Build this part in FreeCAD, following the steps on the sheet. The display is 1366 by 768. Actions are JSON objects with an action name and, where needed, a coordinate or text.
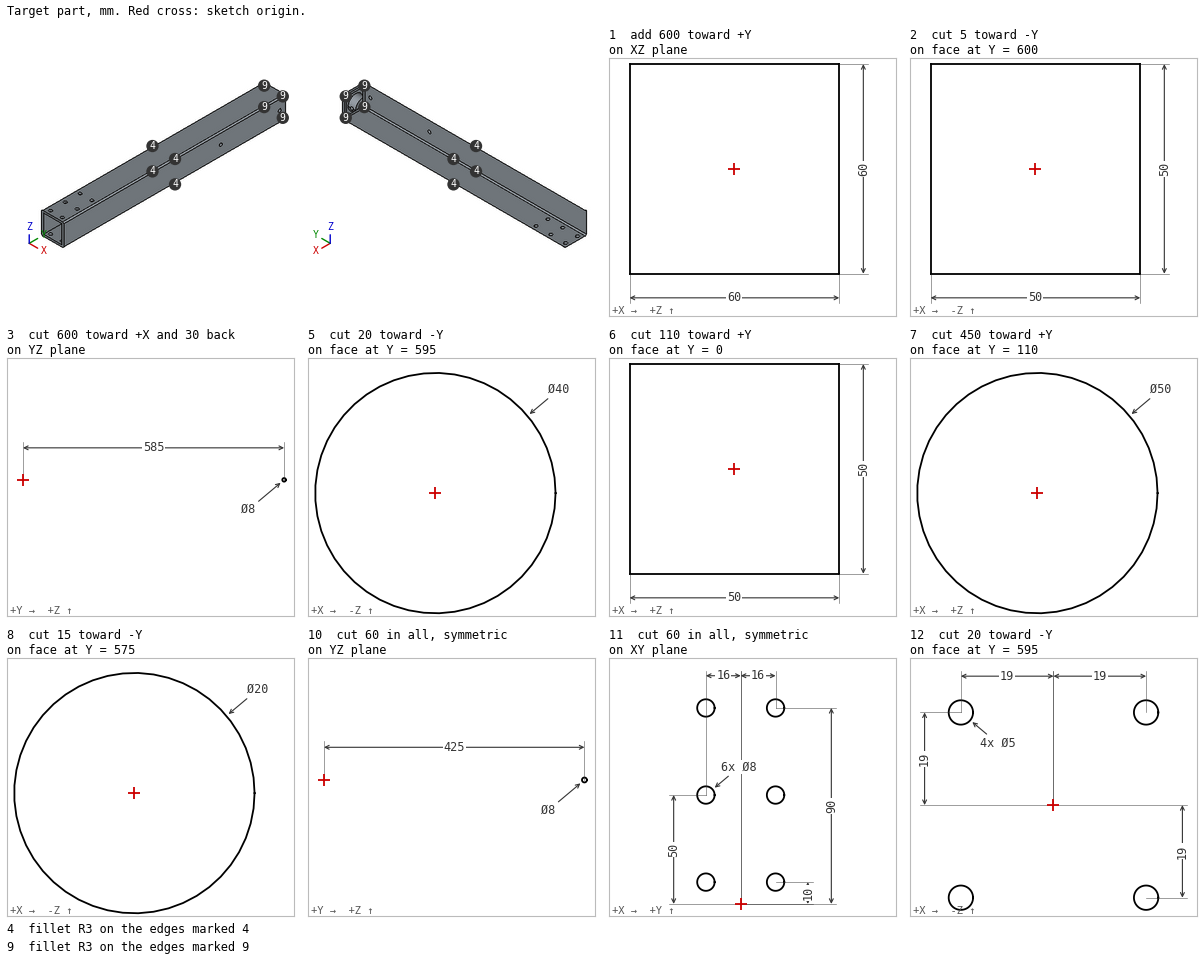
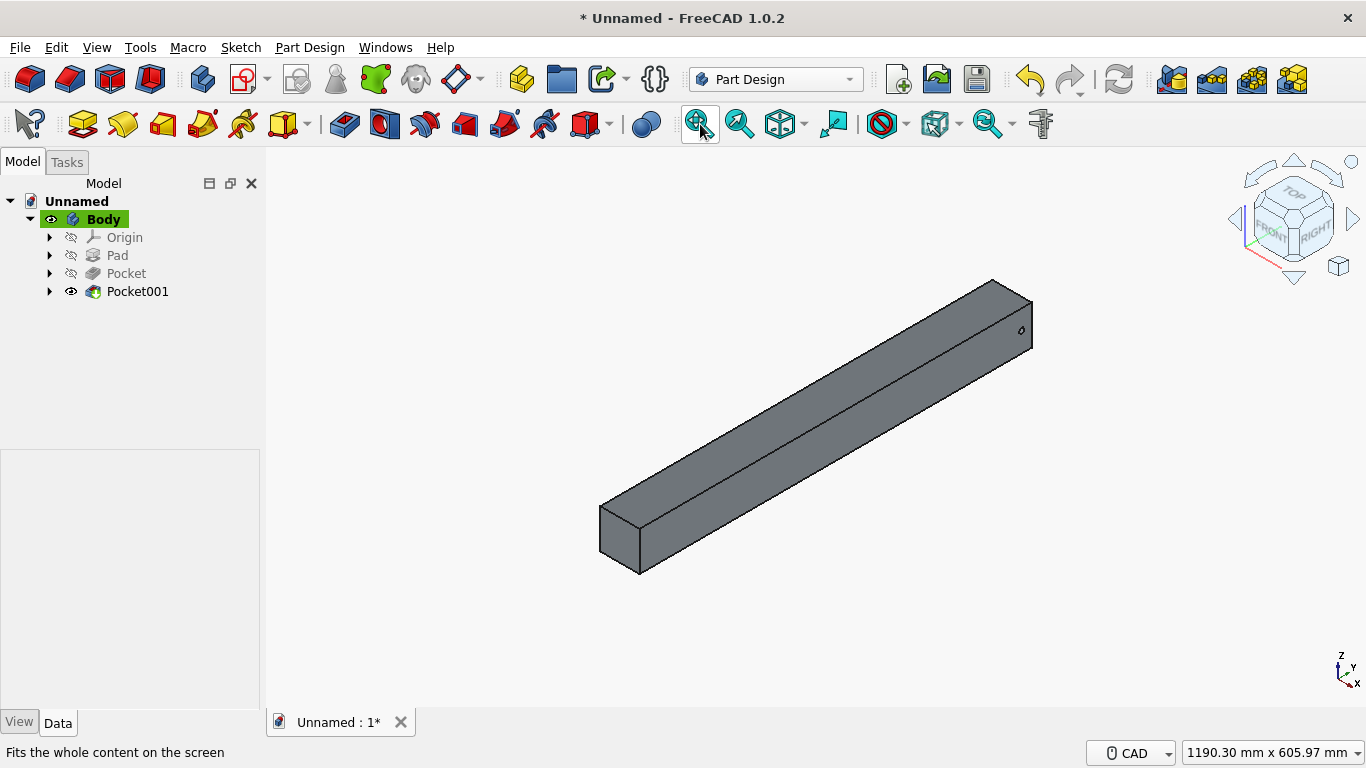
{"action": "left_click", "coordinate": [836, 415]}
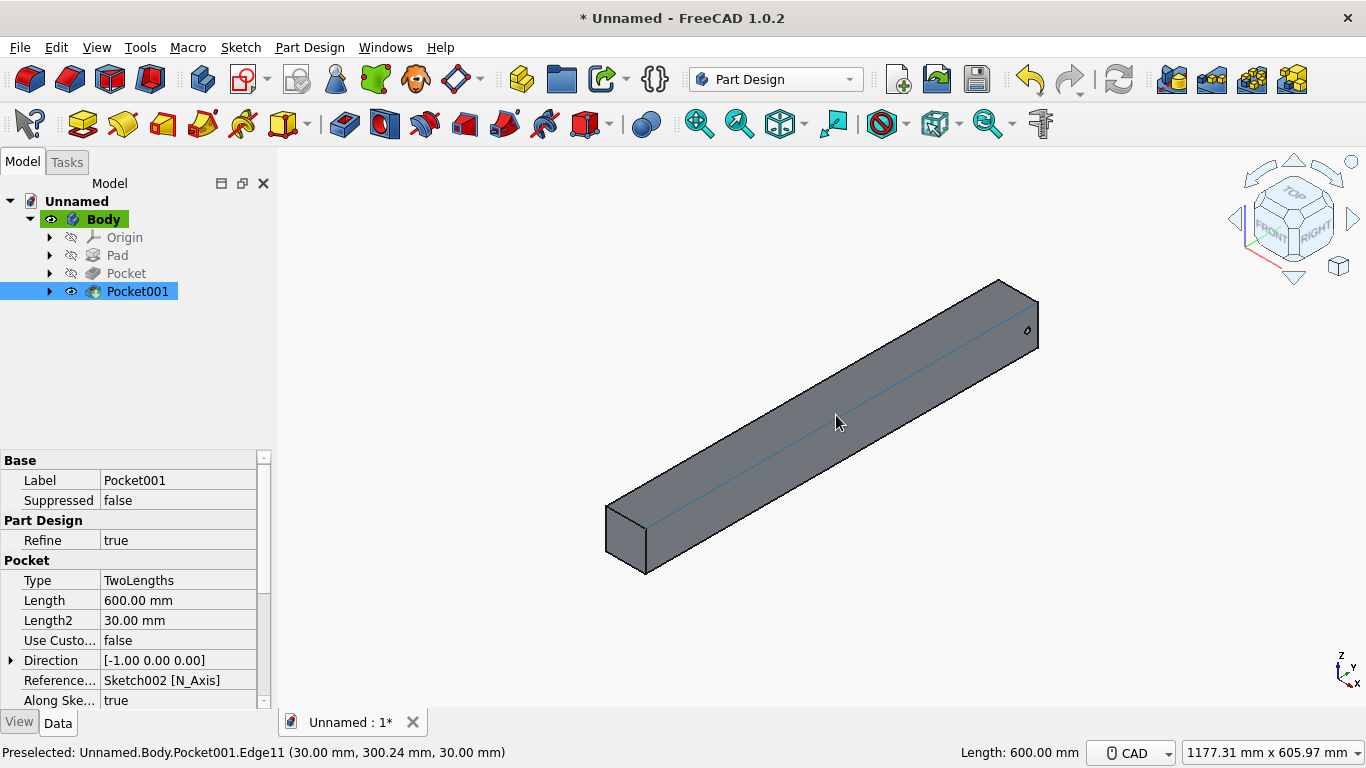
{"action": "key", "text": "2"}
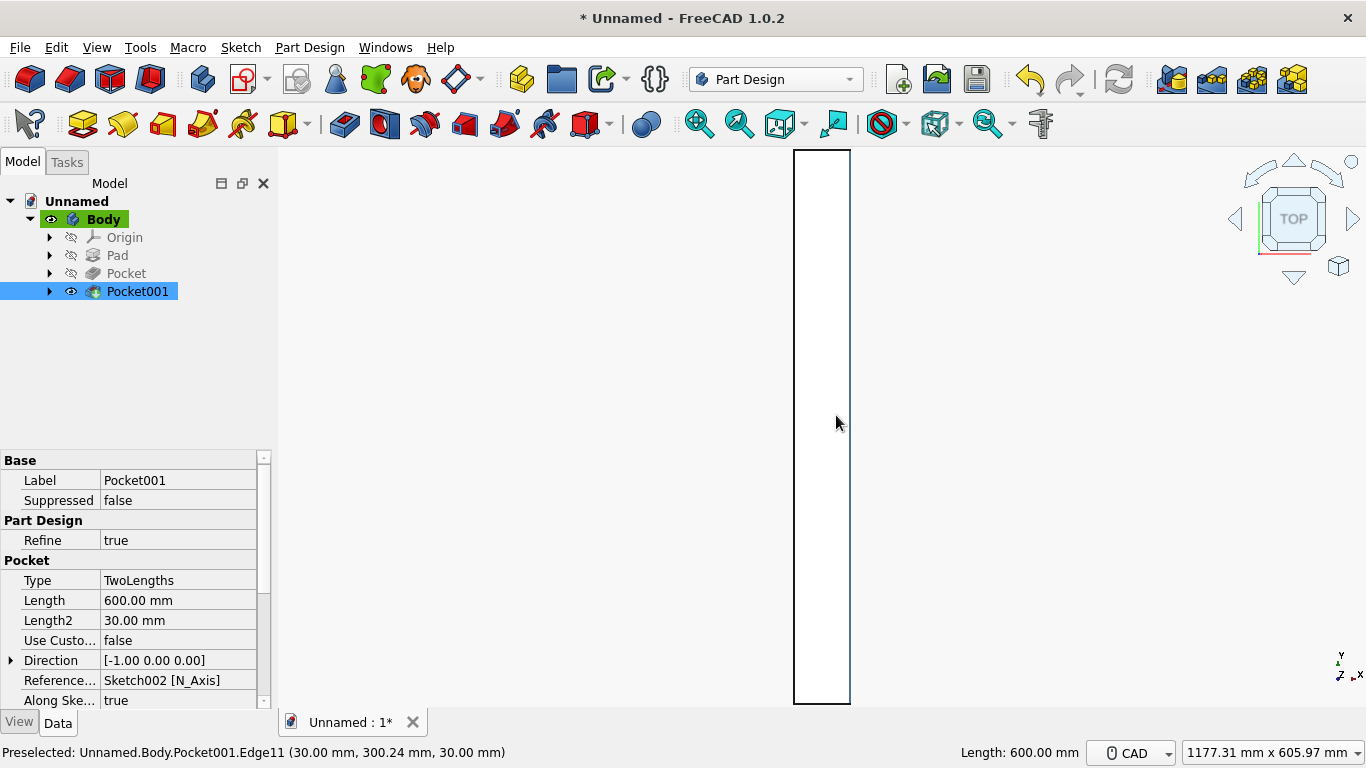
{"action": "left_click", "coordinate": [794, 426], "text": "ctrl"}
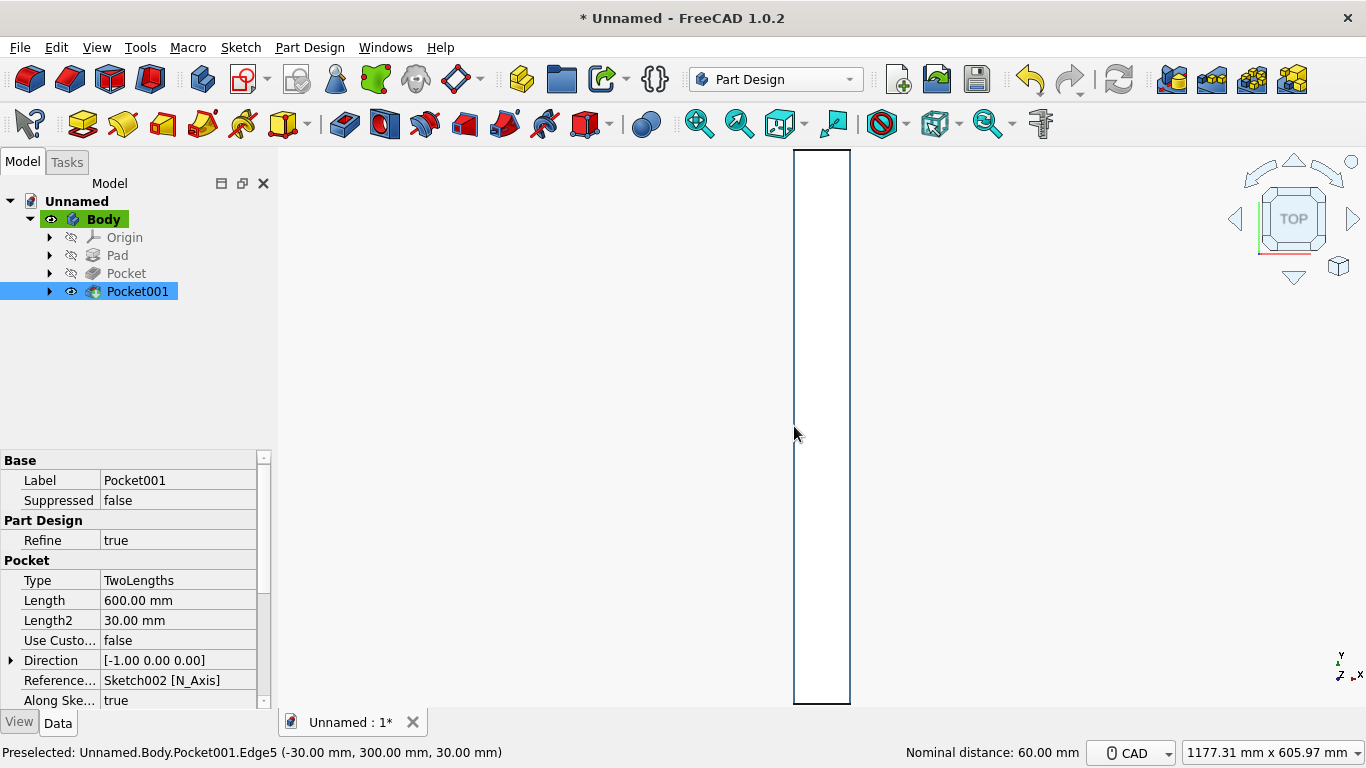
{"action": "key", "text": "1"}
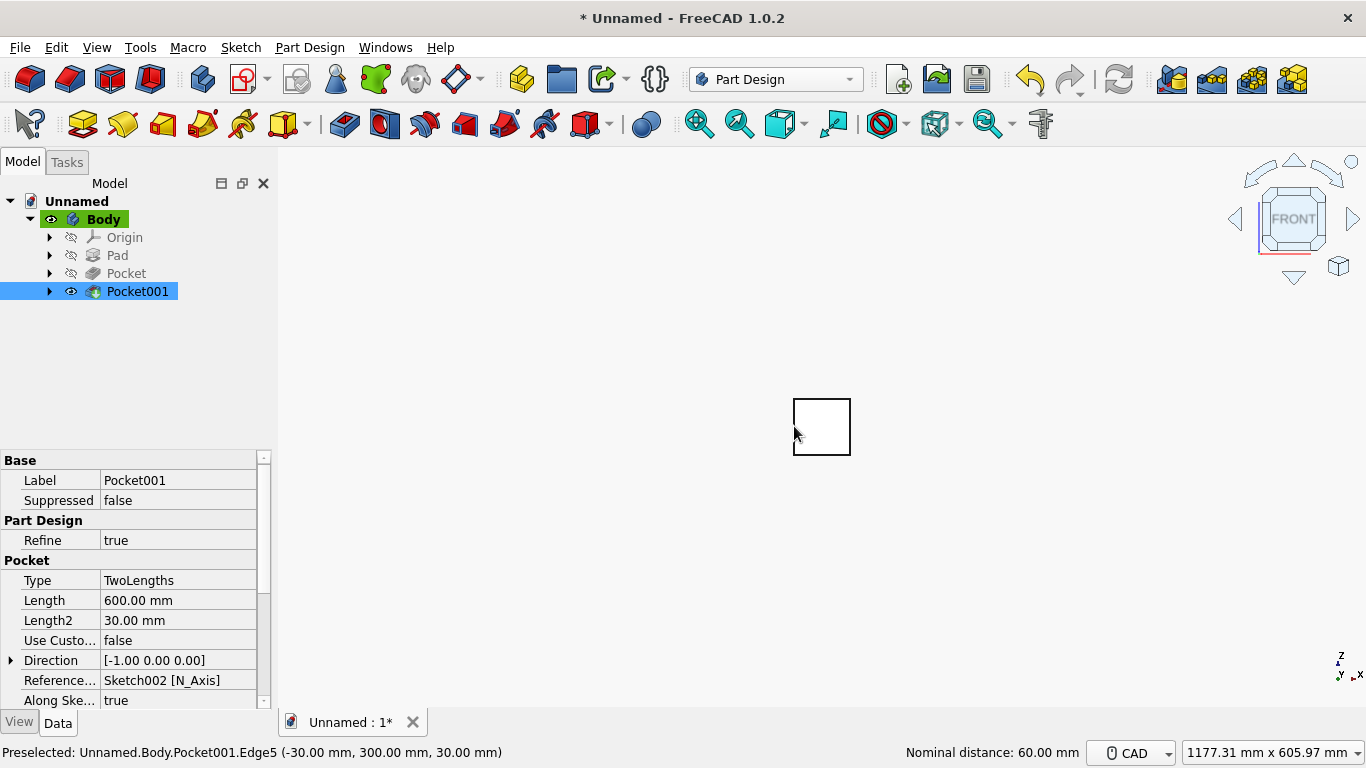
{"action": "left_click", "coordinate": [700, 124]}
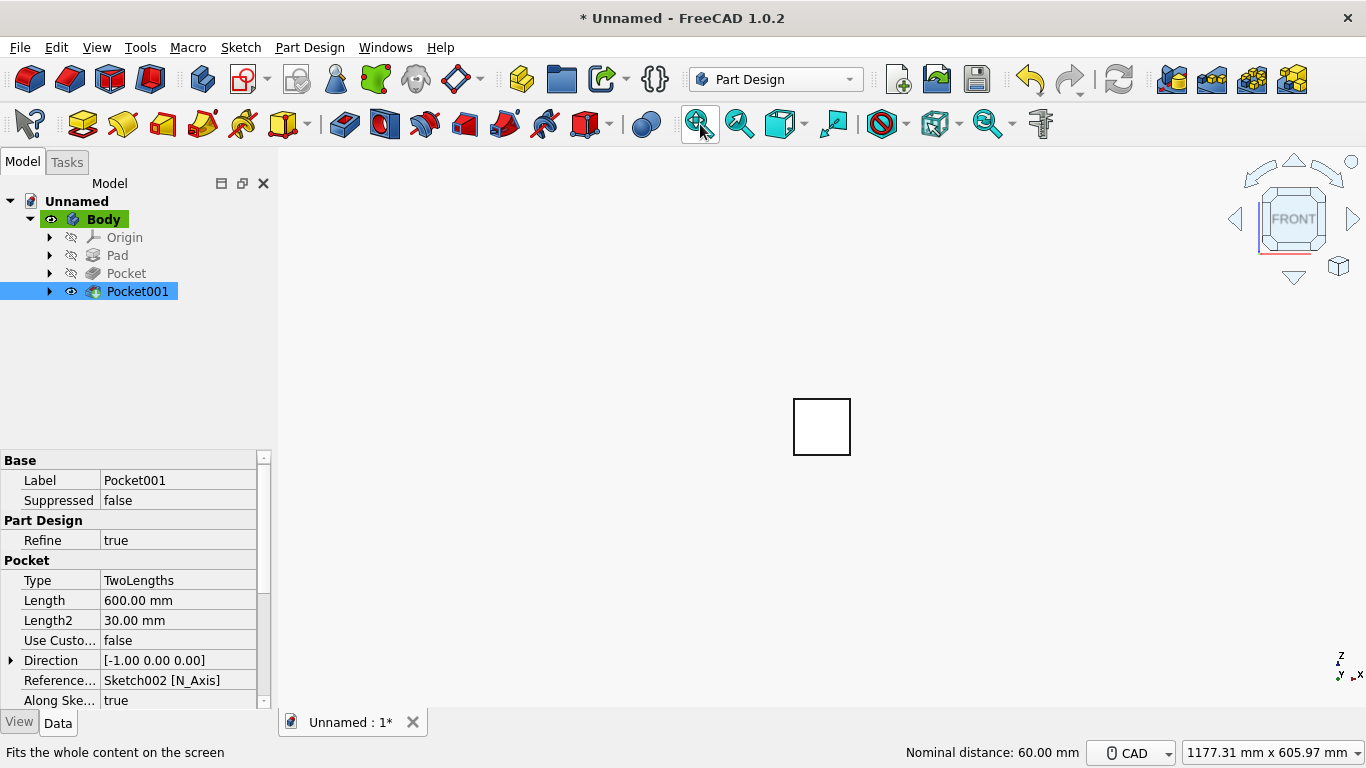
{"action": "key", "text": "3"}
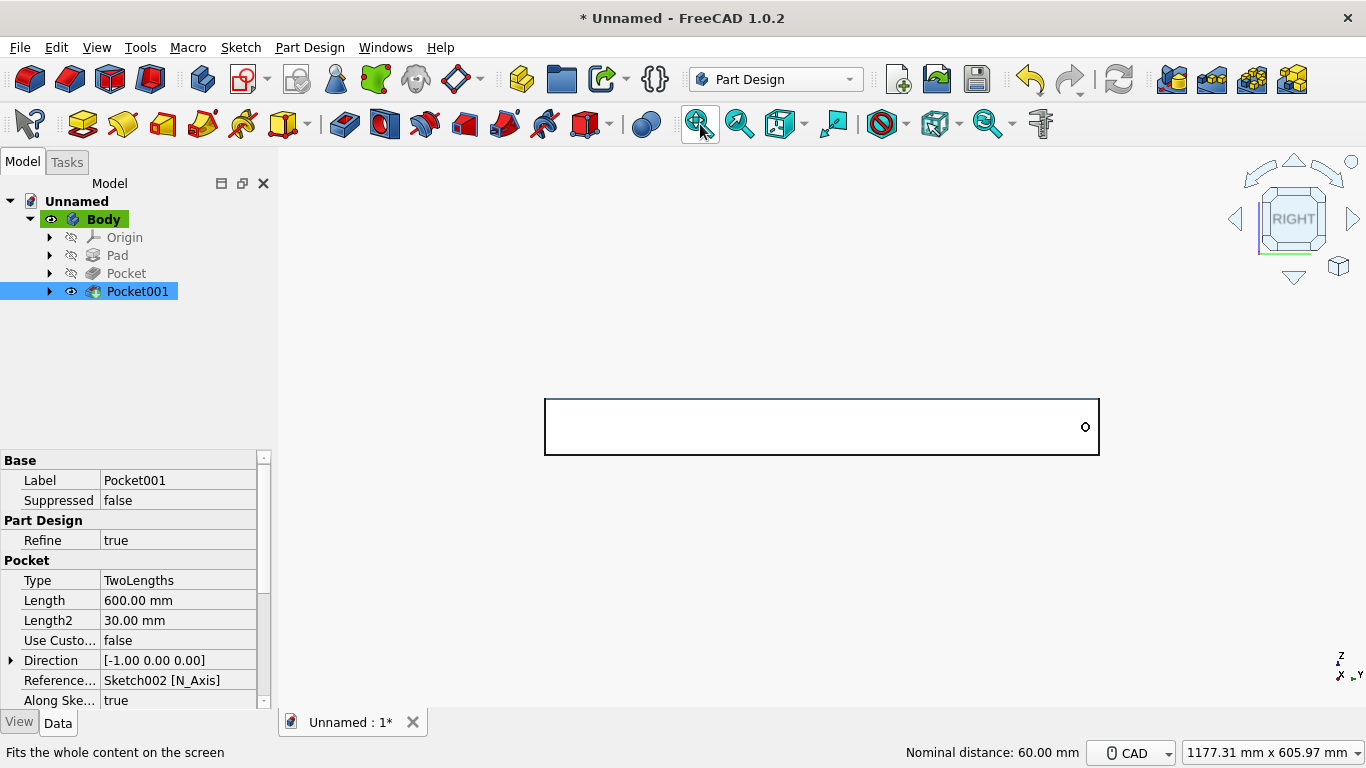
{"action": "left_click", "coordinate": [822, 454], "text": "ctrl"}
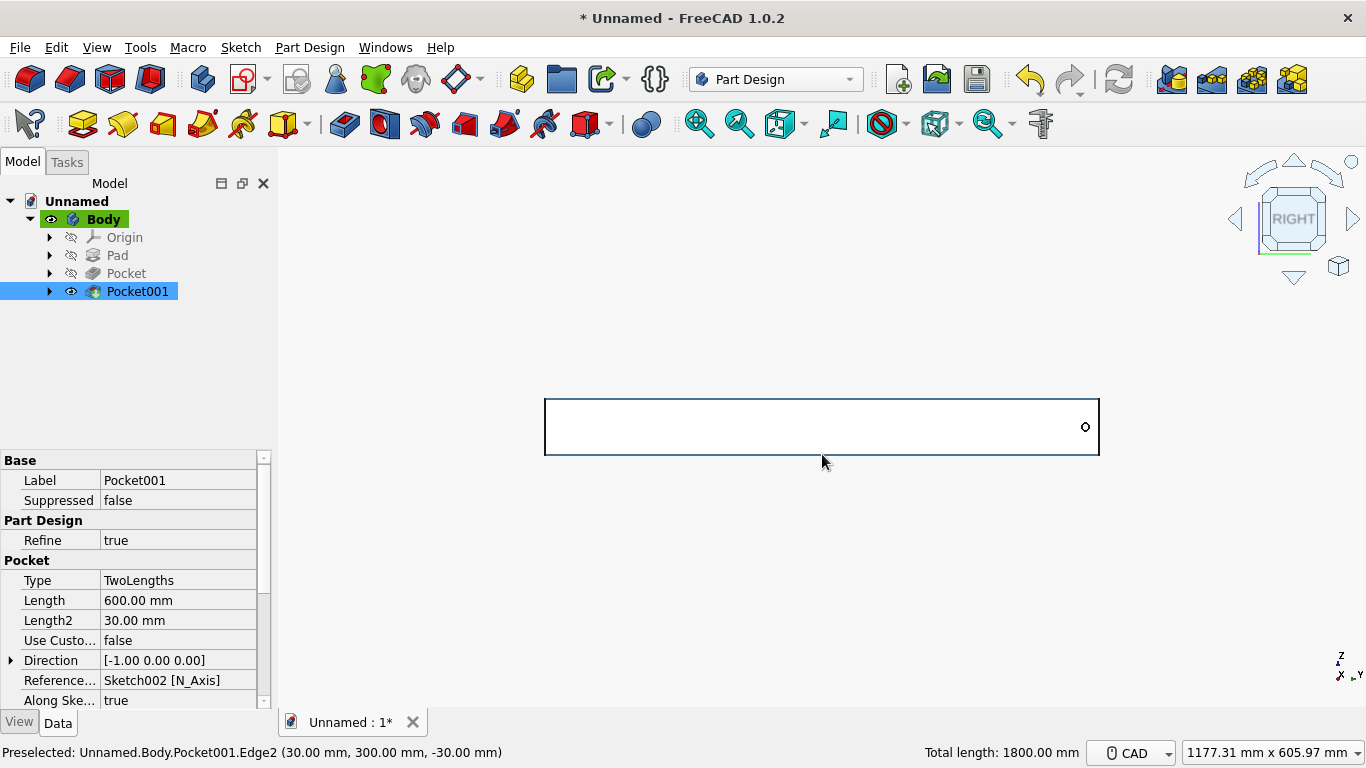
{"action": "key", "text": "5"}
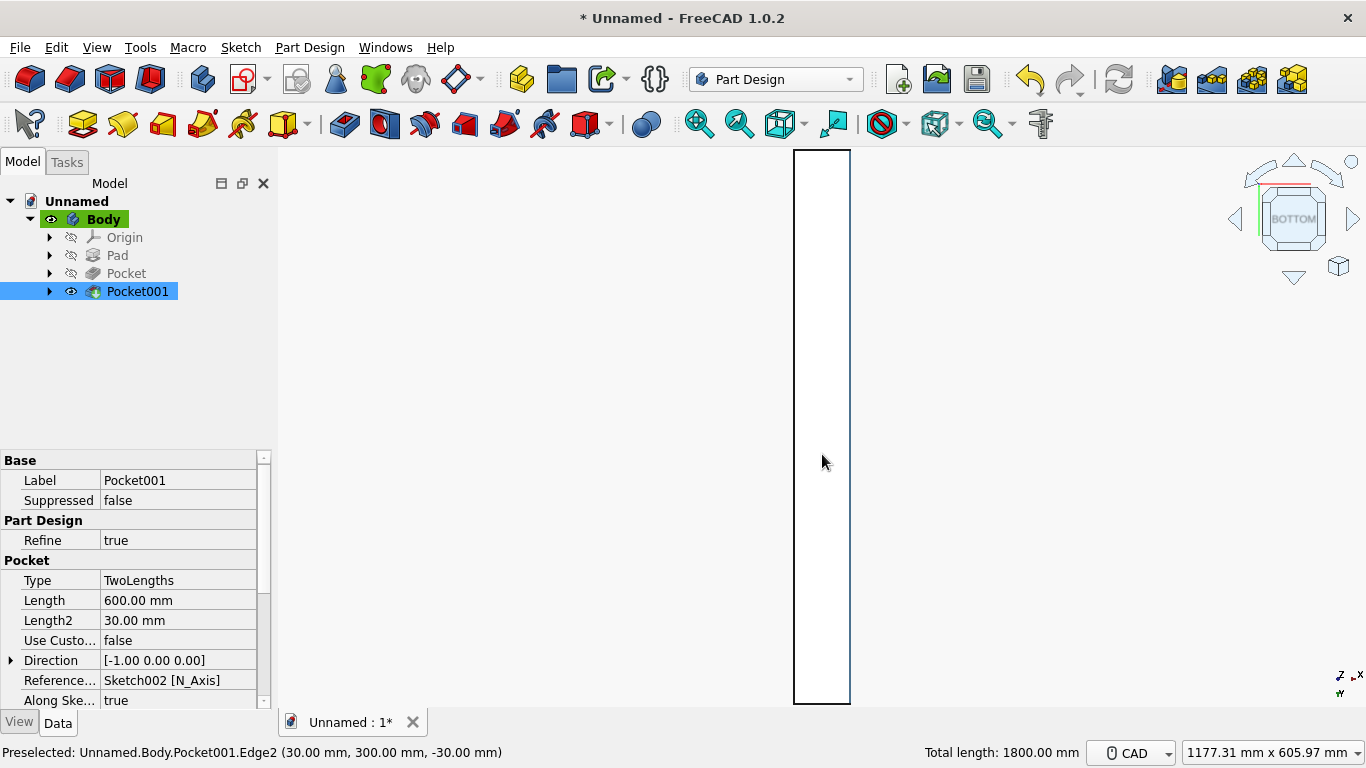
{"action": "left_click", "coordinate": [794, 426], "text": "ctrl"}